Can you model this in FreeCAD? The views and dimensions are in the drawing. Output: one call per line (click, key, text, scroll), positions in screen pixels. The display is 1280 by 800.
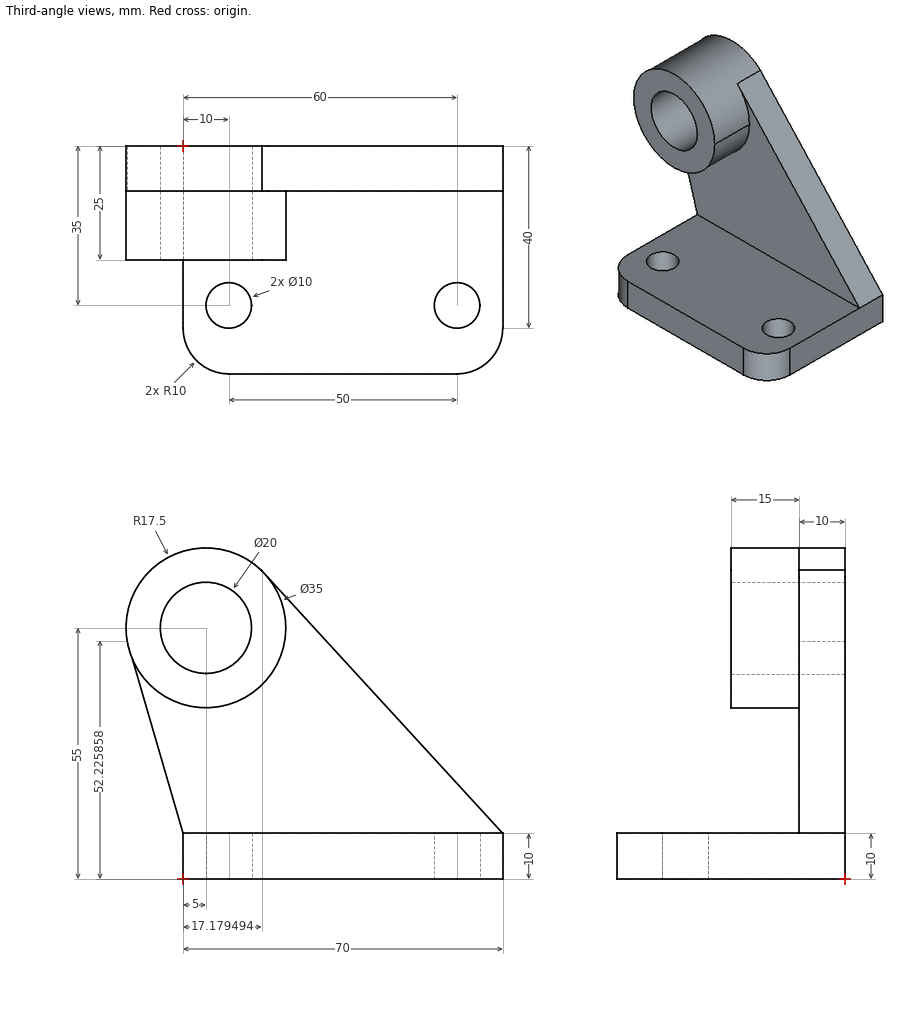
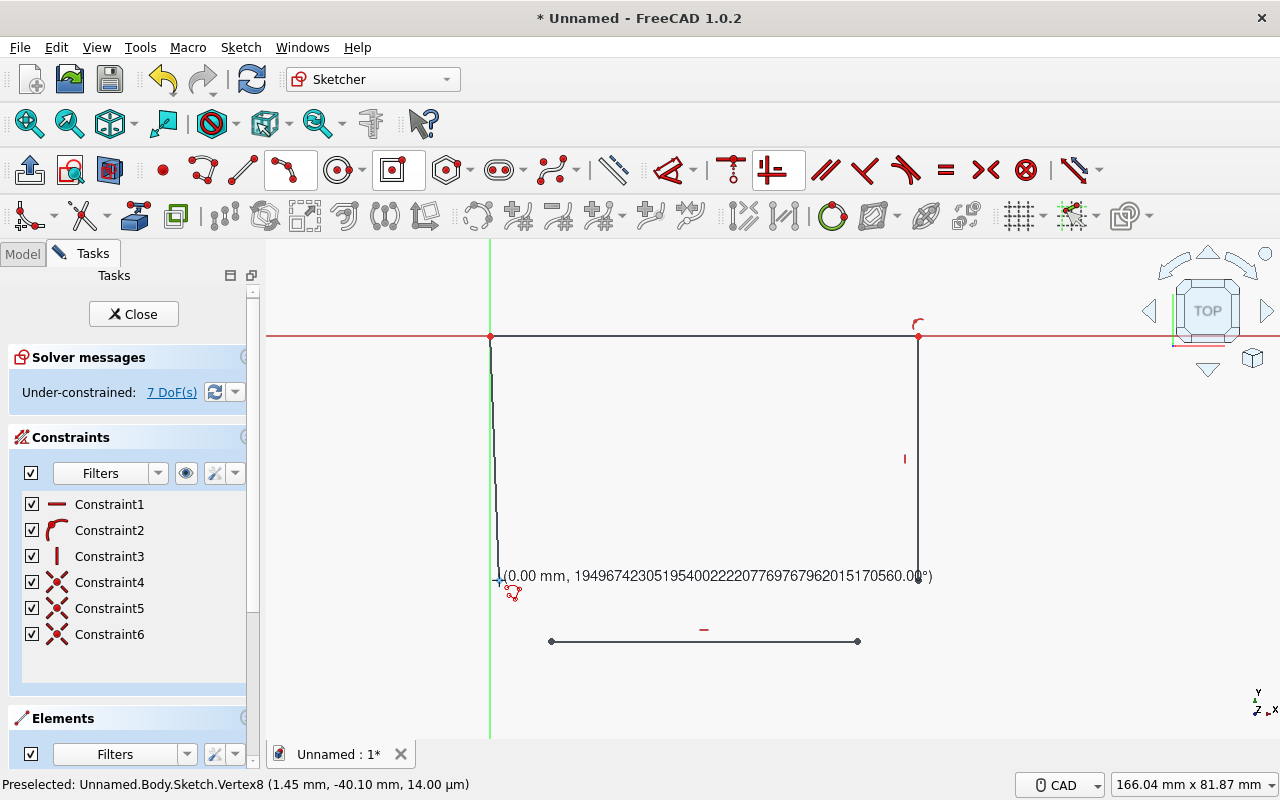
click(284, 170)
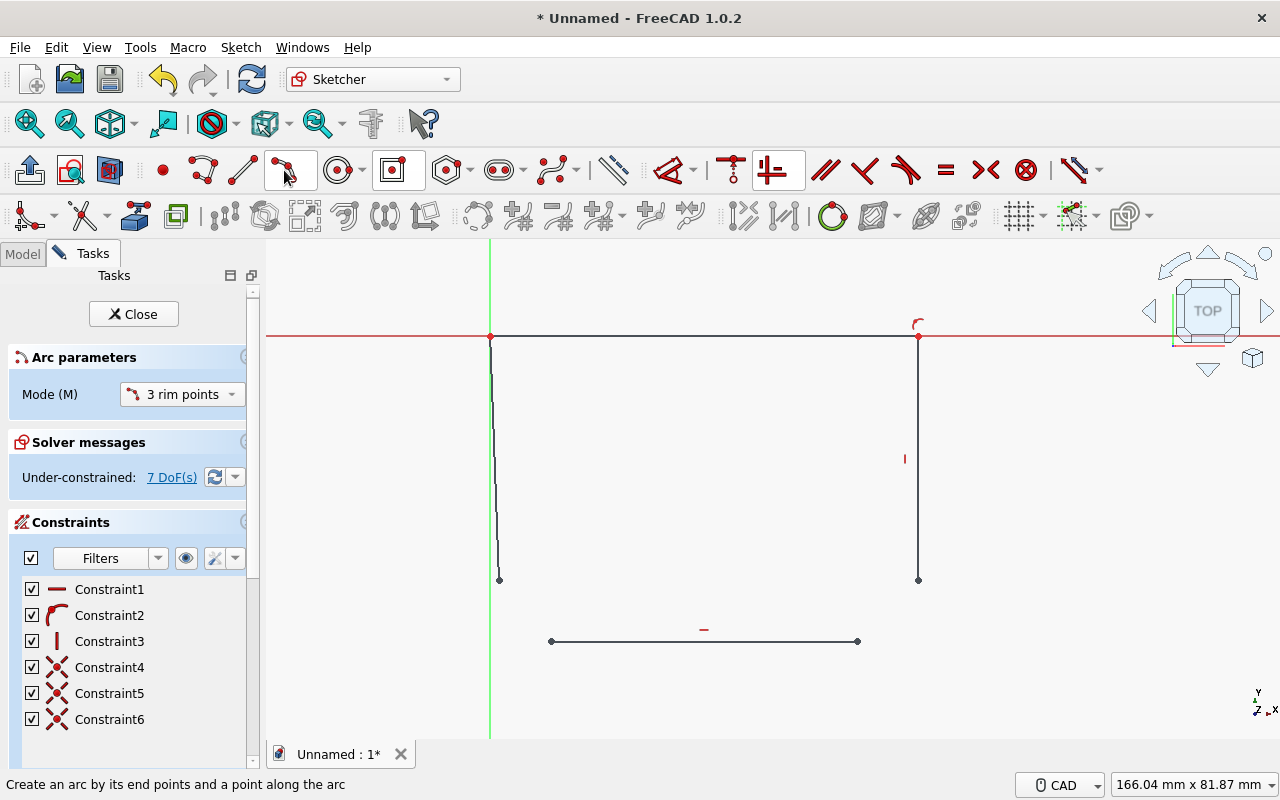
click(857, 642)
click(918, 581)
click(900, 624)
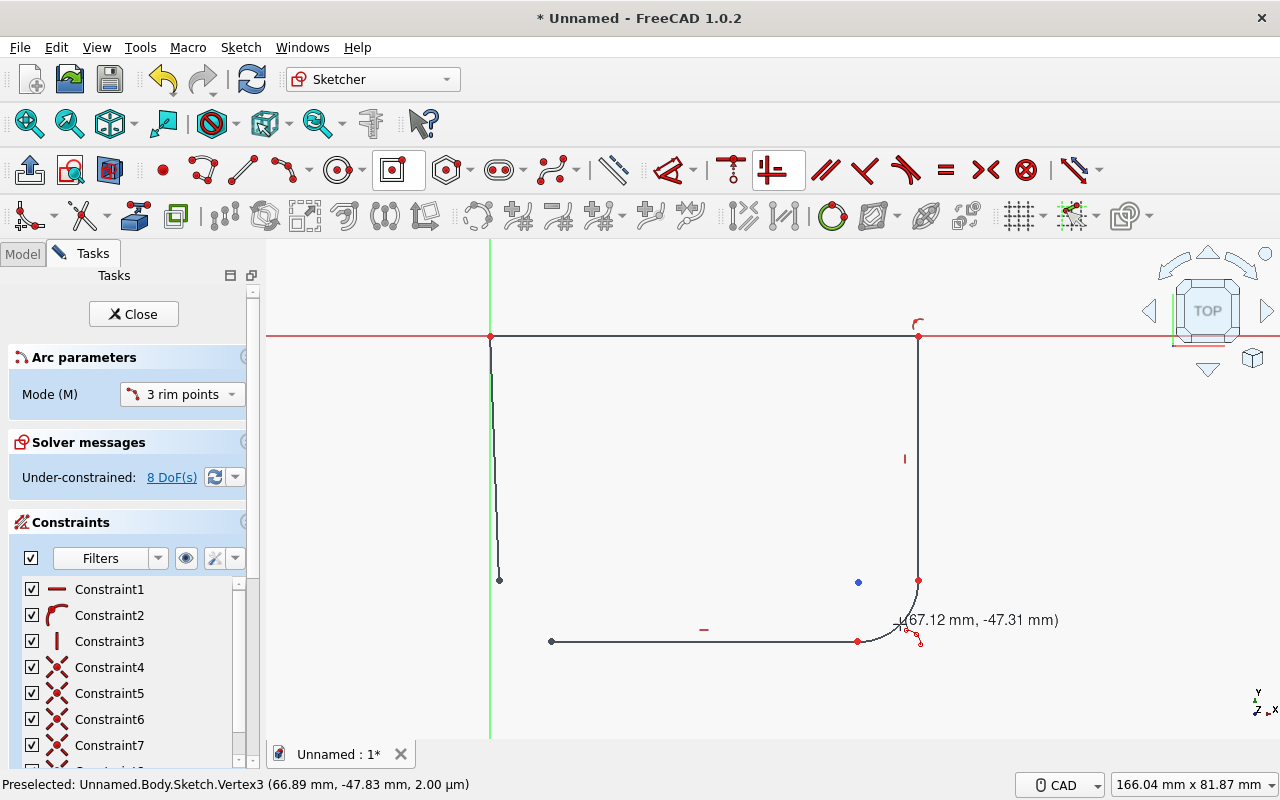
click(499, 581)
click(551, 642)
click(508, 624)
key(Escape)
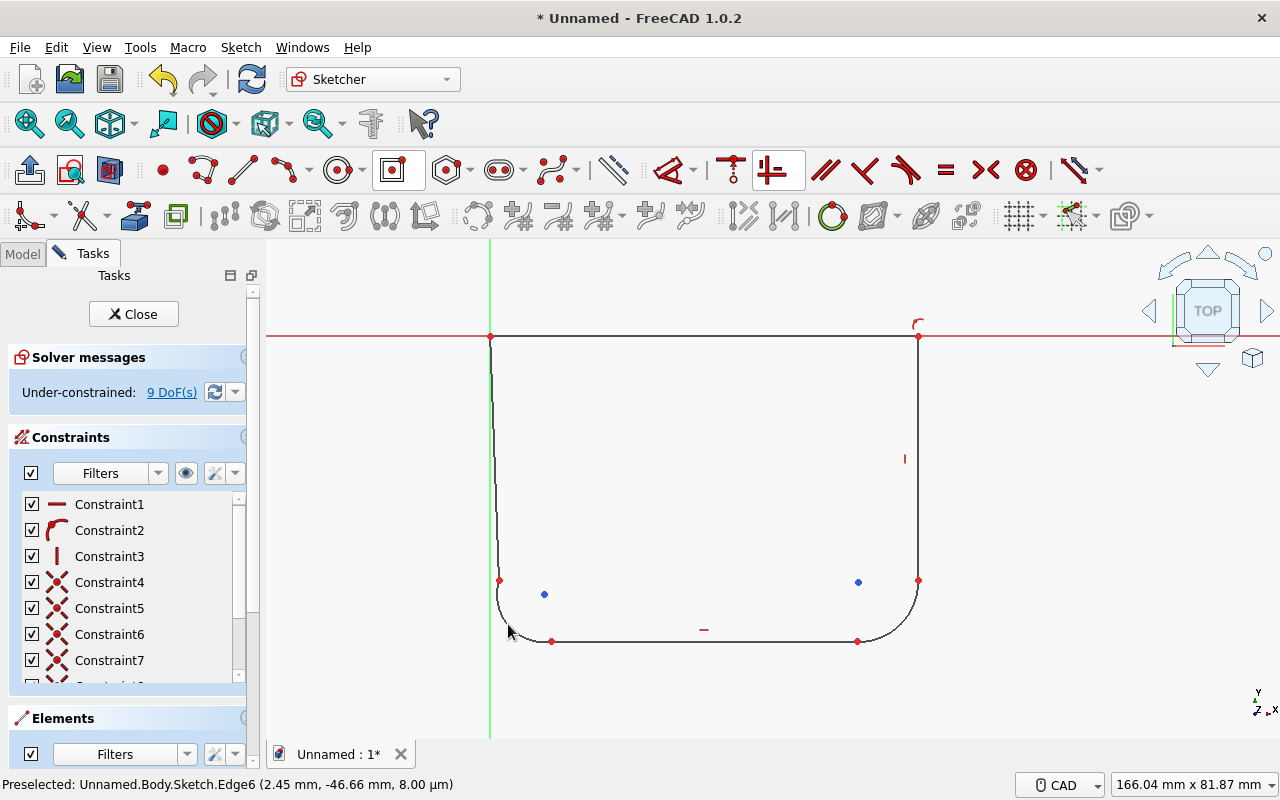
click(643, 642)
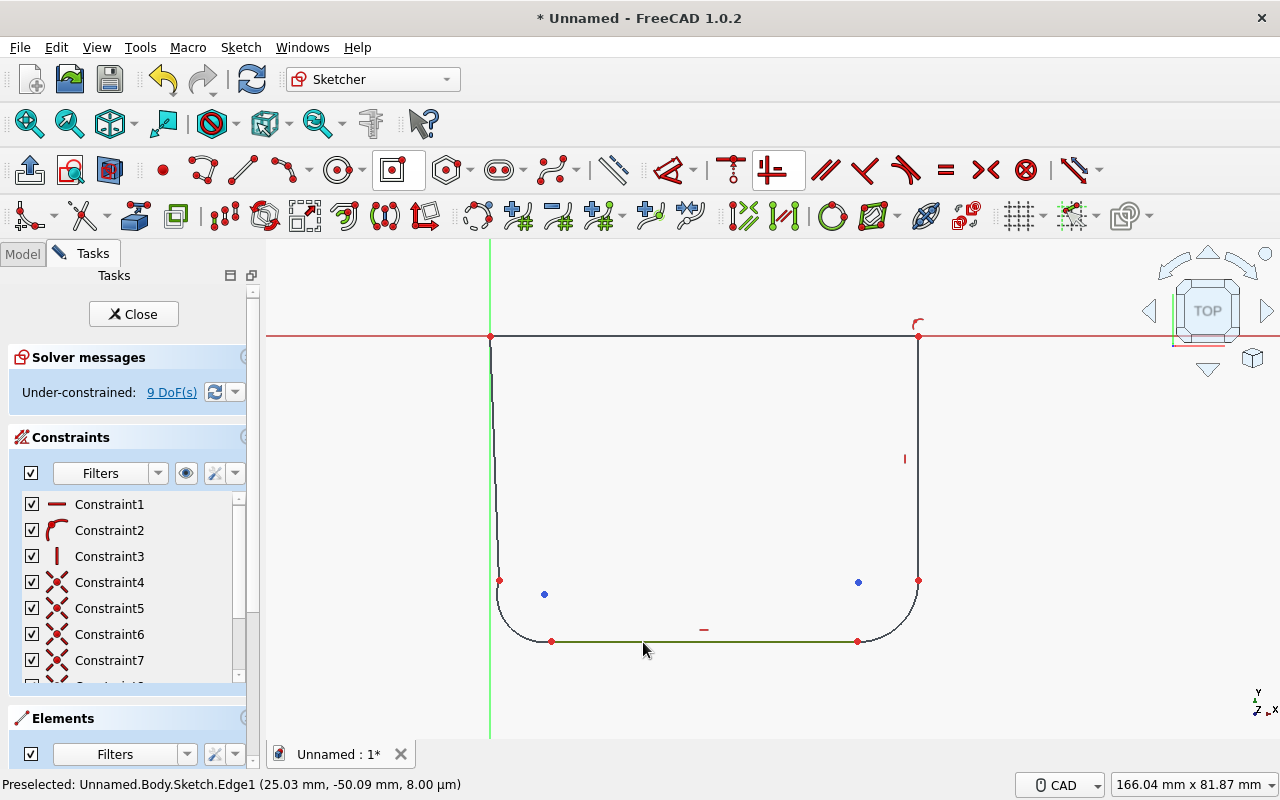
click(885, 636)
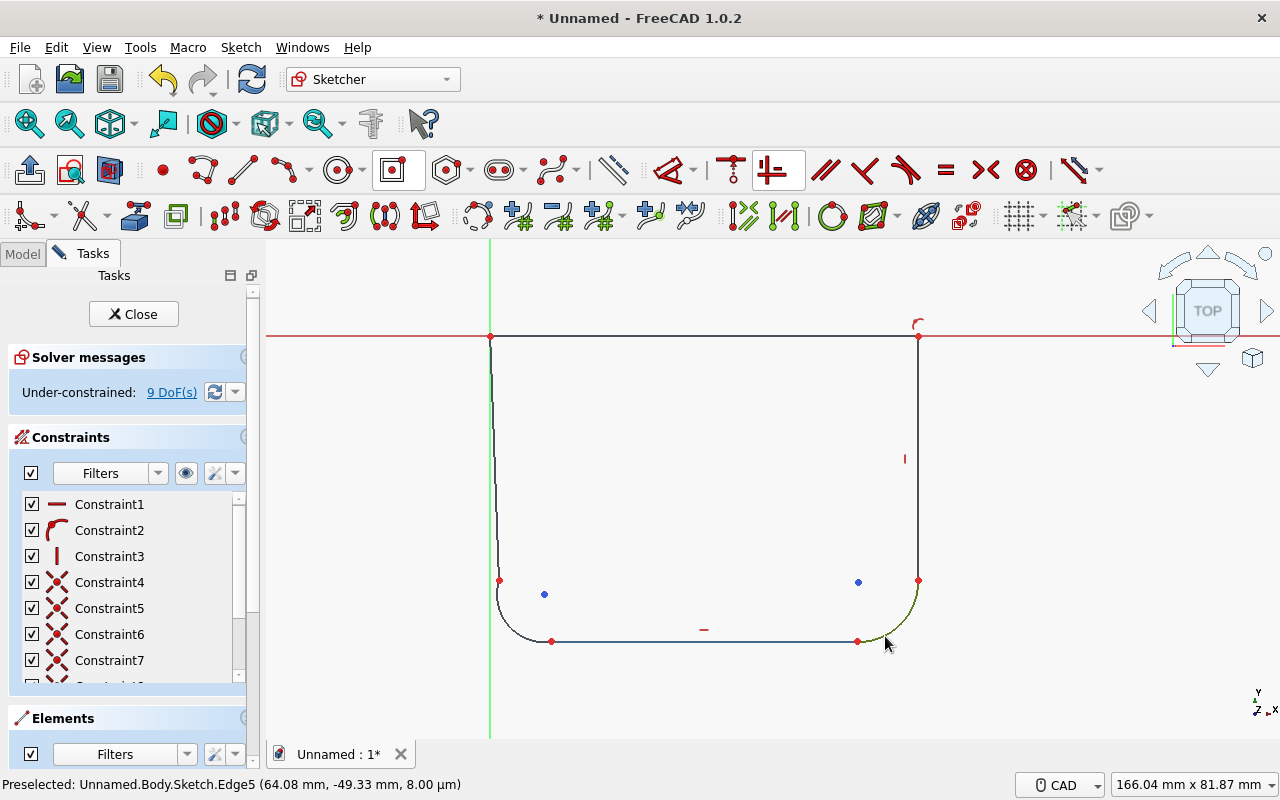
key(t)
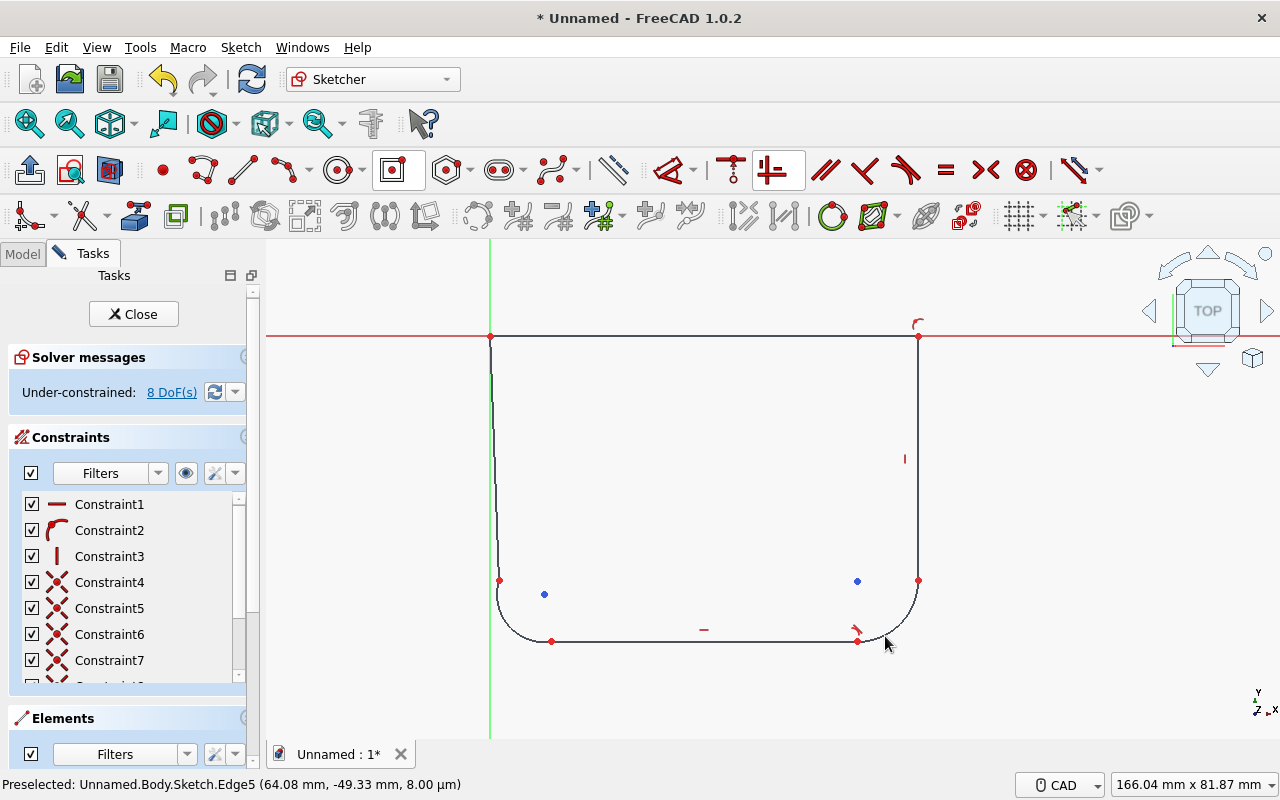
click(643, 642)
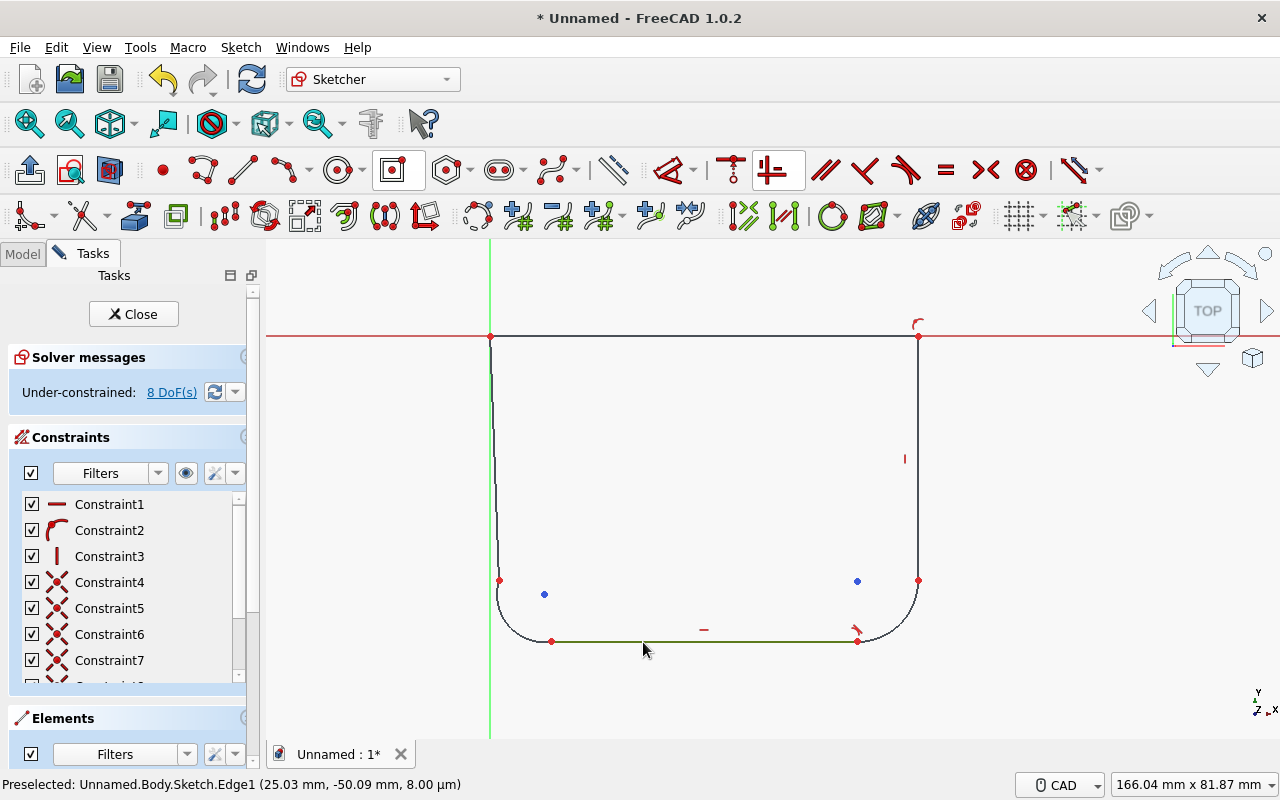
scroll(499, 609, up, 3)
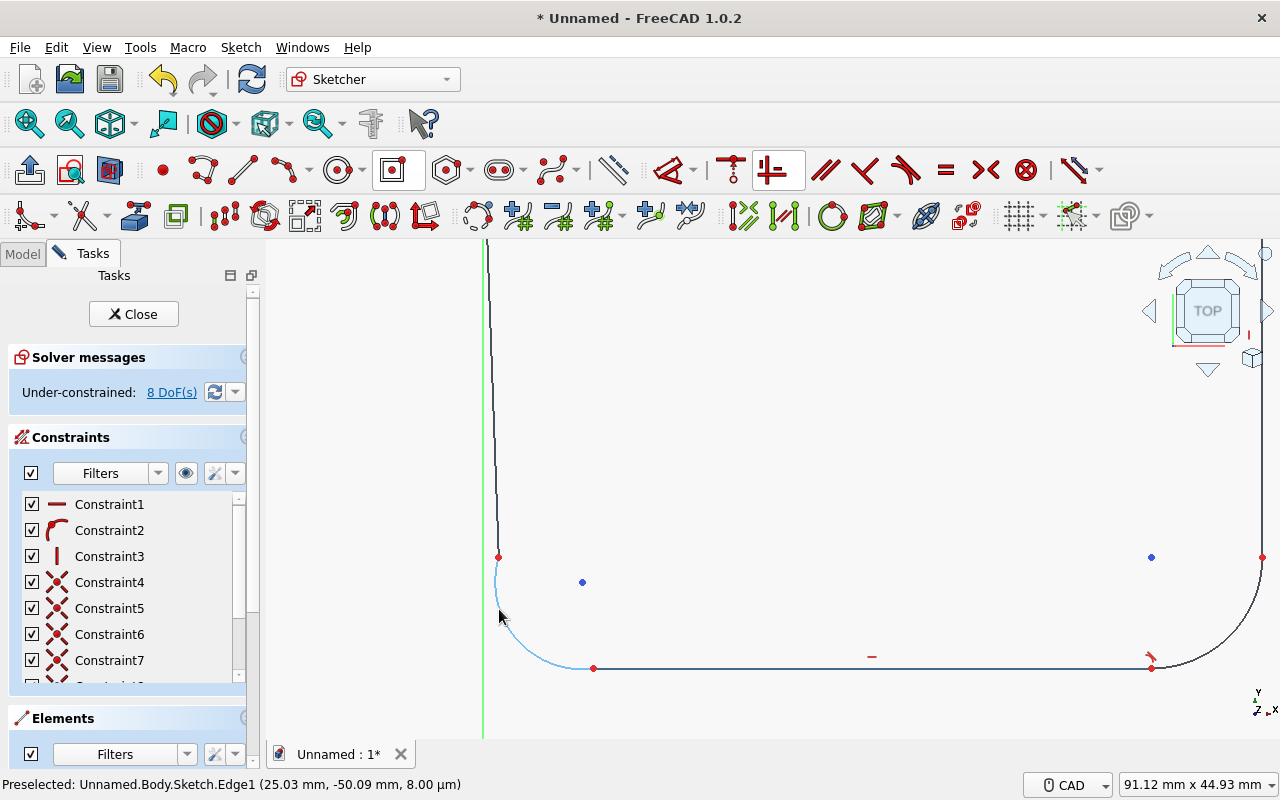
click(499, 609)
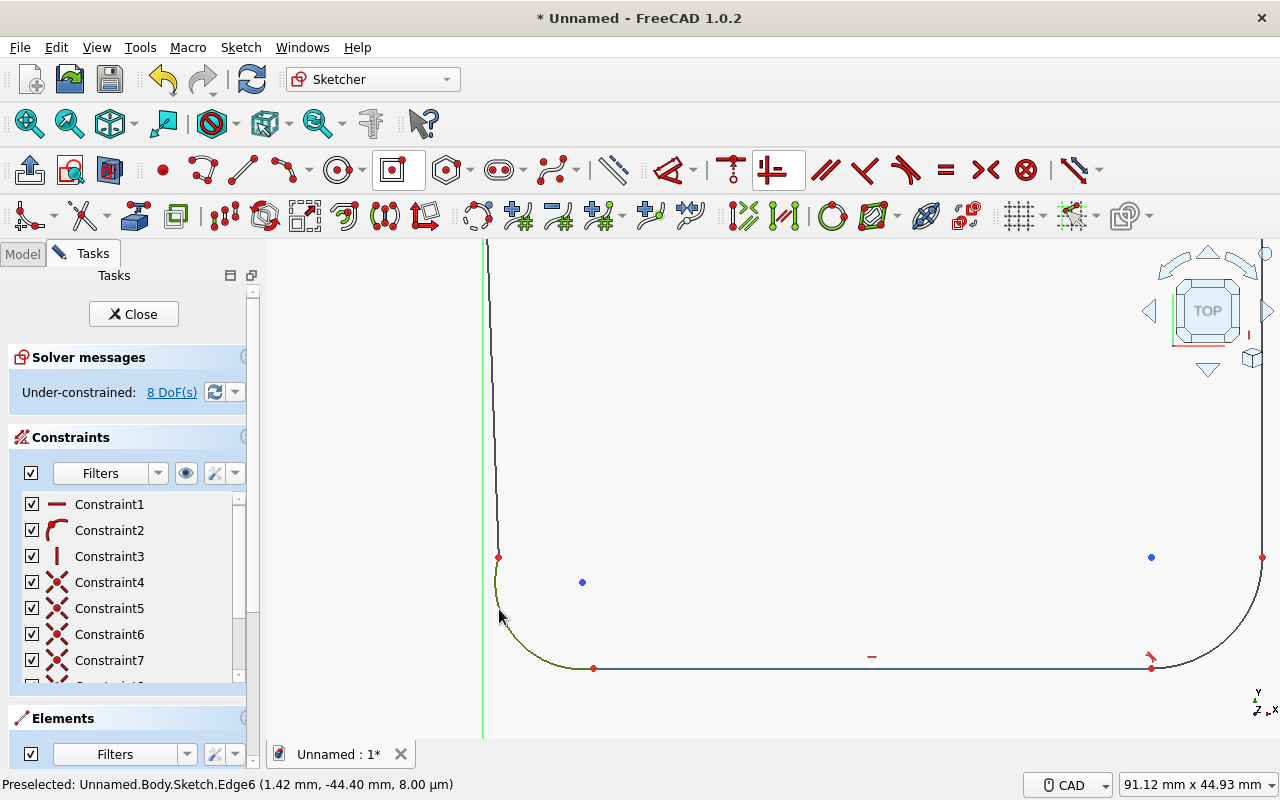
click(906, 170)